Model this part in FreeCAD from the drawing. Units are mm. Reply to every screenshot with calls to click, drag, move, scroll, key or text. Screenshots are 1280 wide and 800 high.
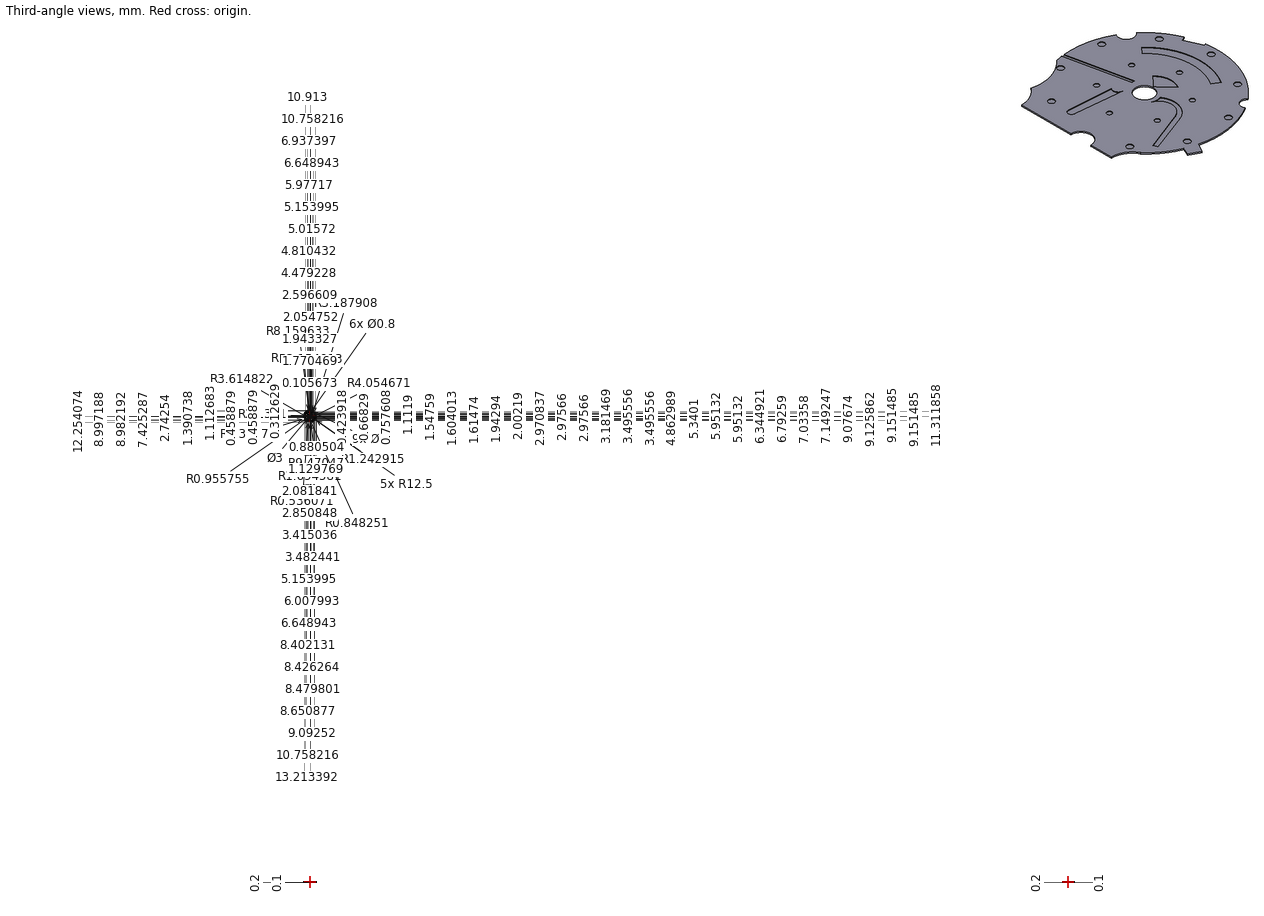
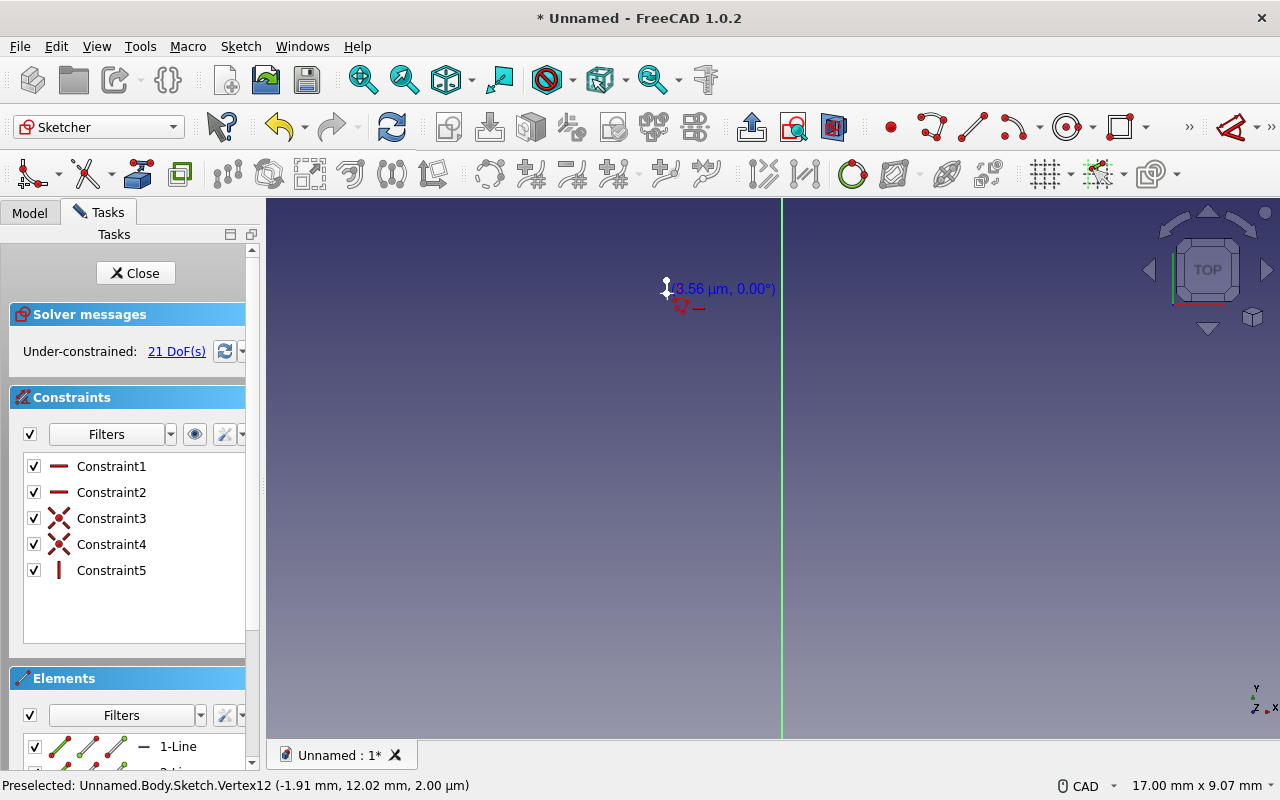
scroll(668, 292, down, 7)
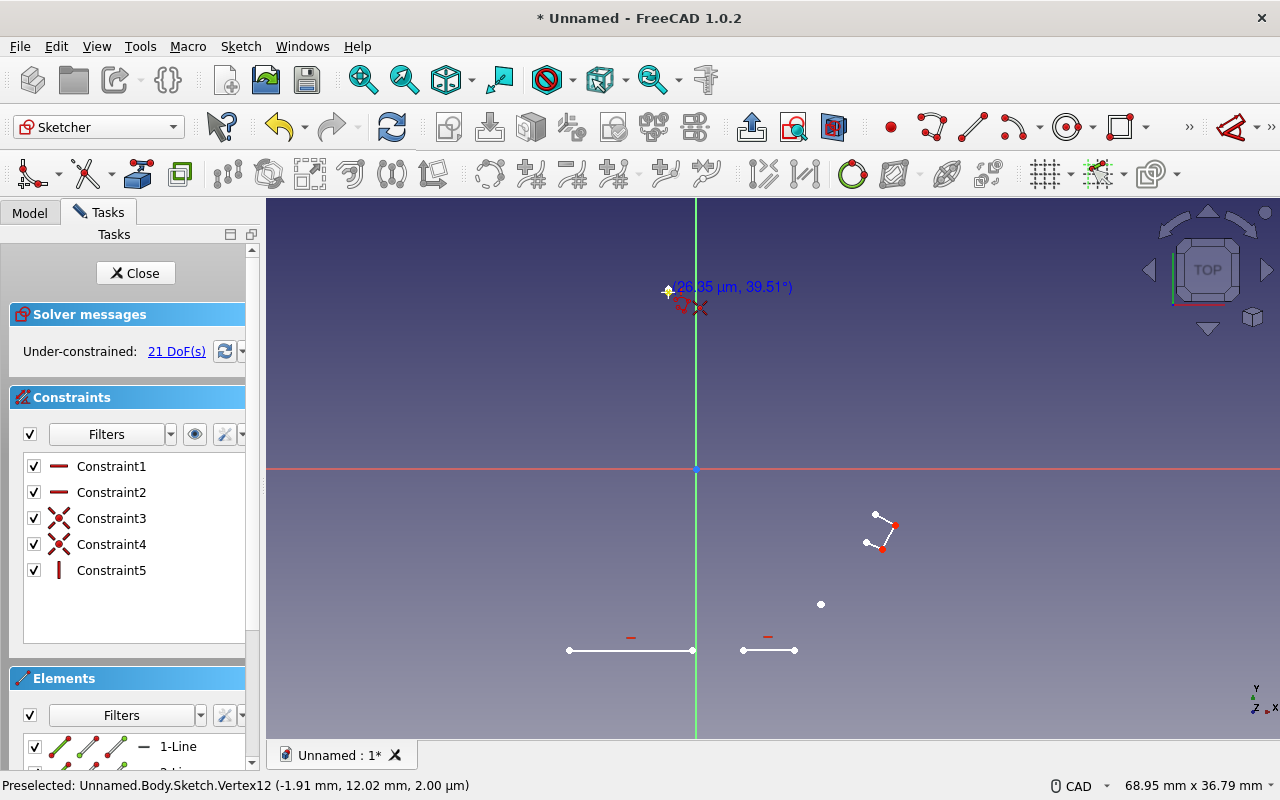
click(630, 309)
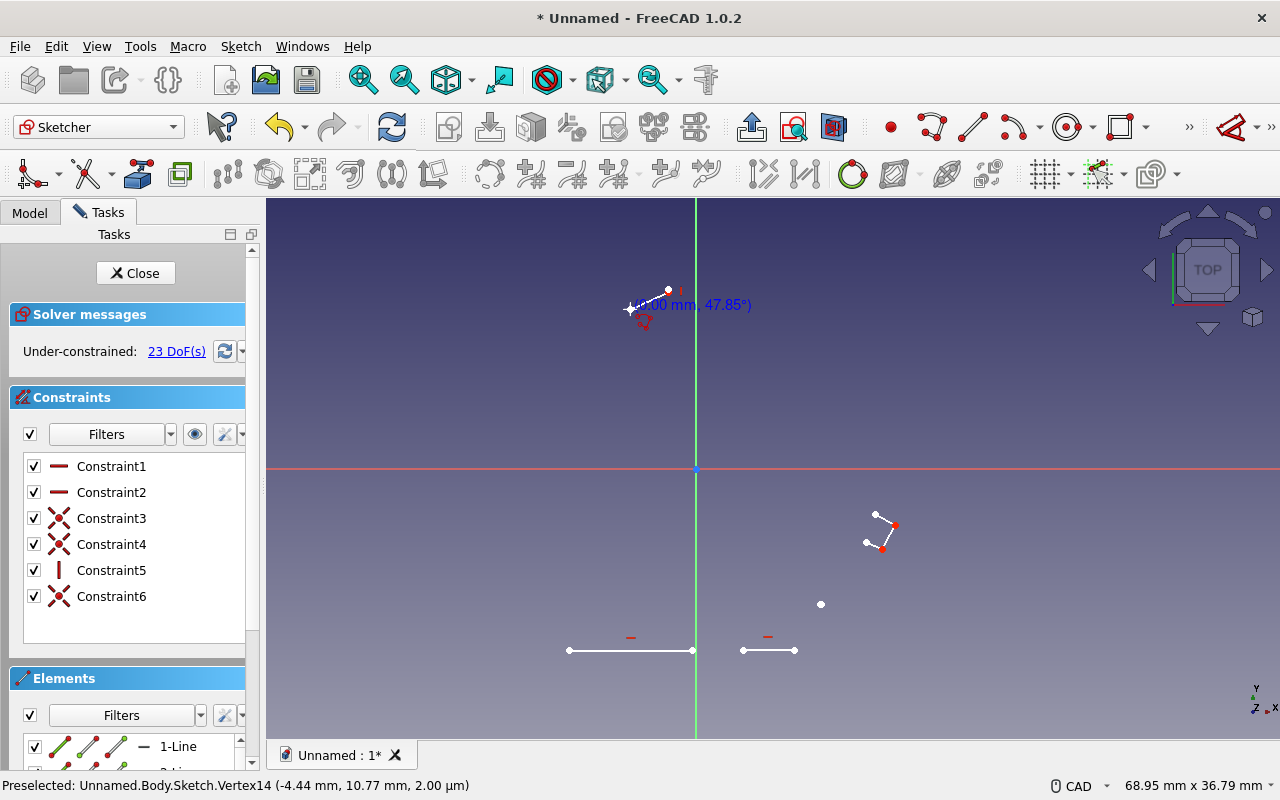
scroll(626, 300, up, 3)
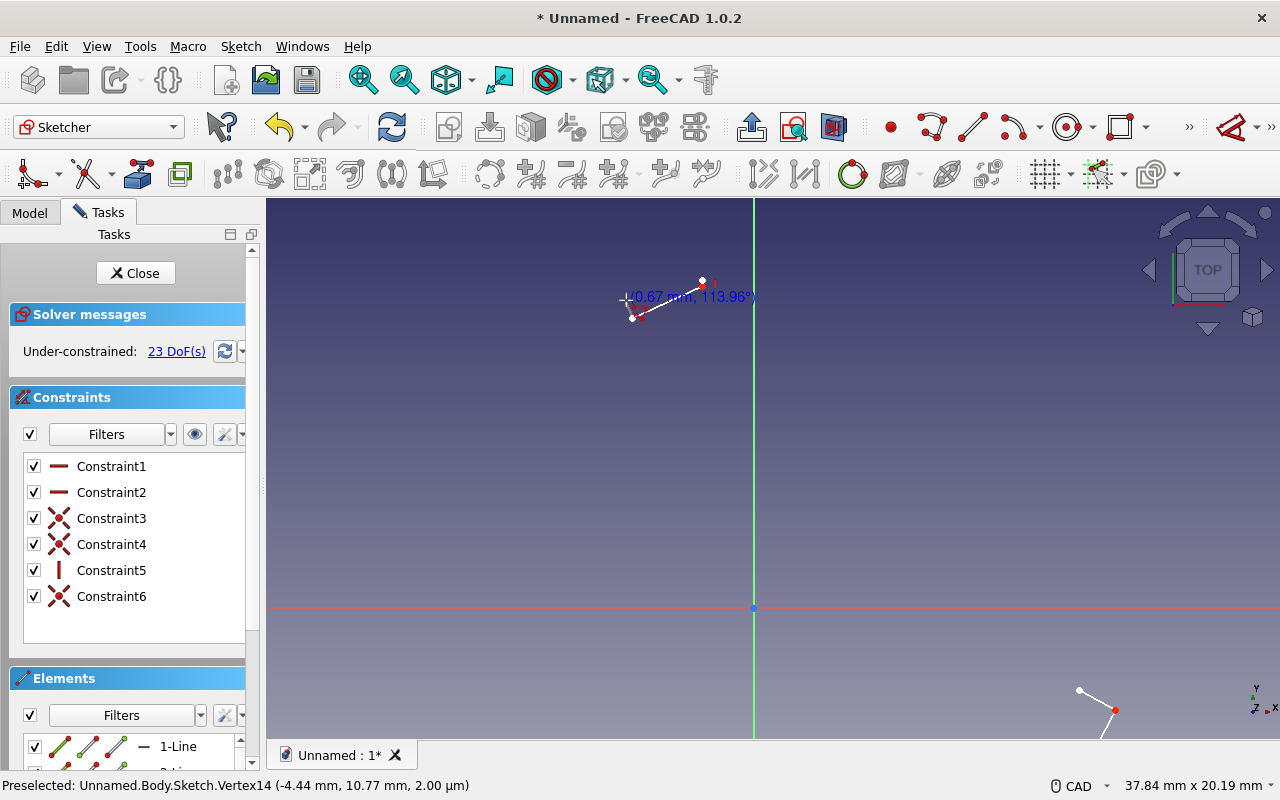
click(625, 299)
right_click(625, 299)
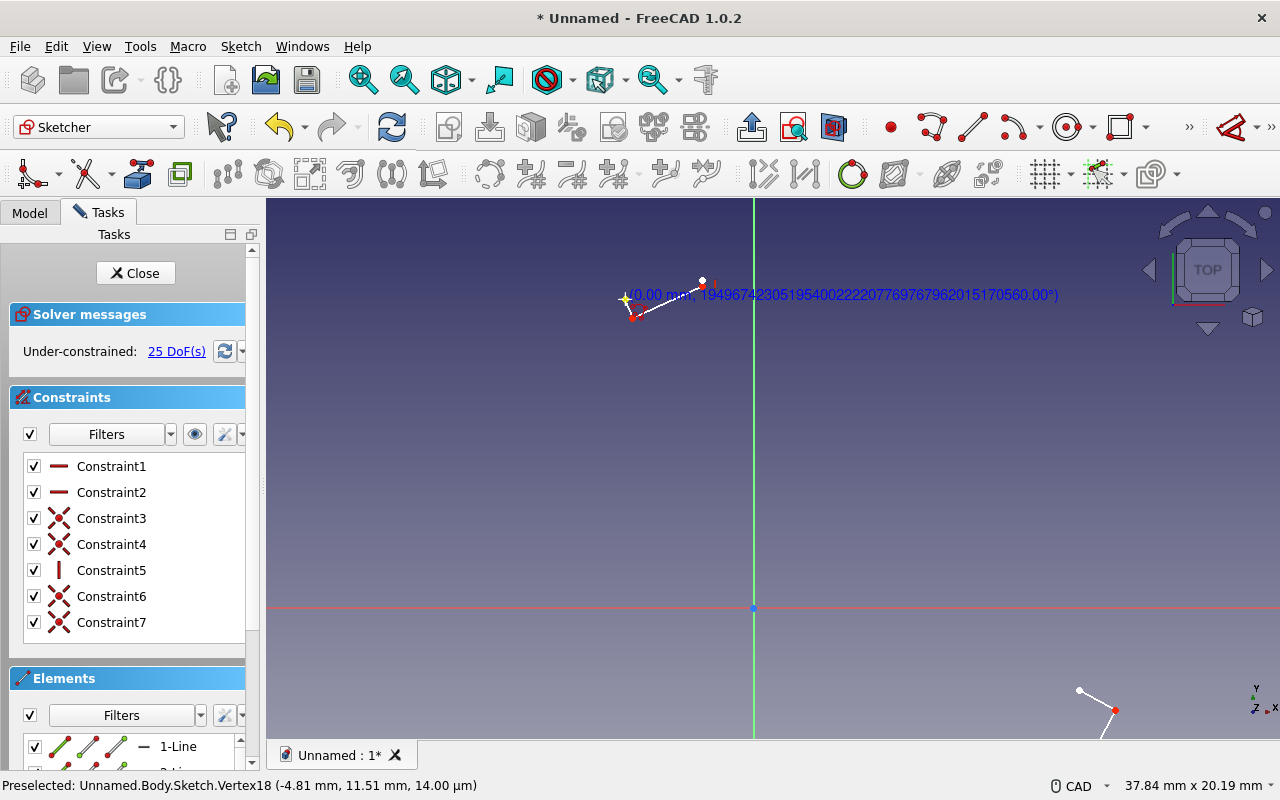
click(1040, 128)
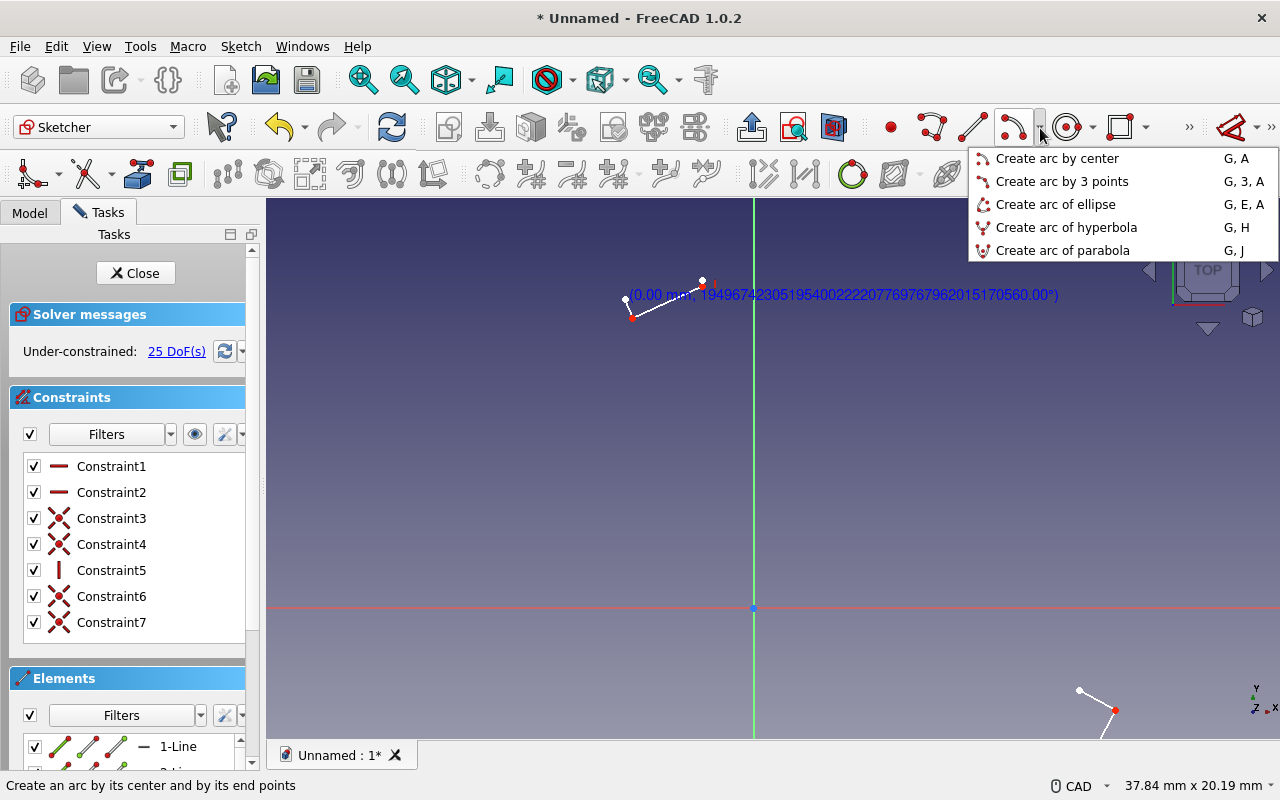
click(1124, 182)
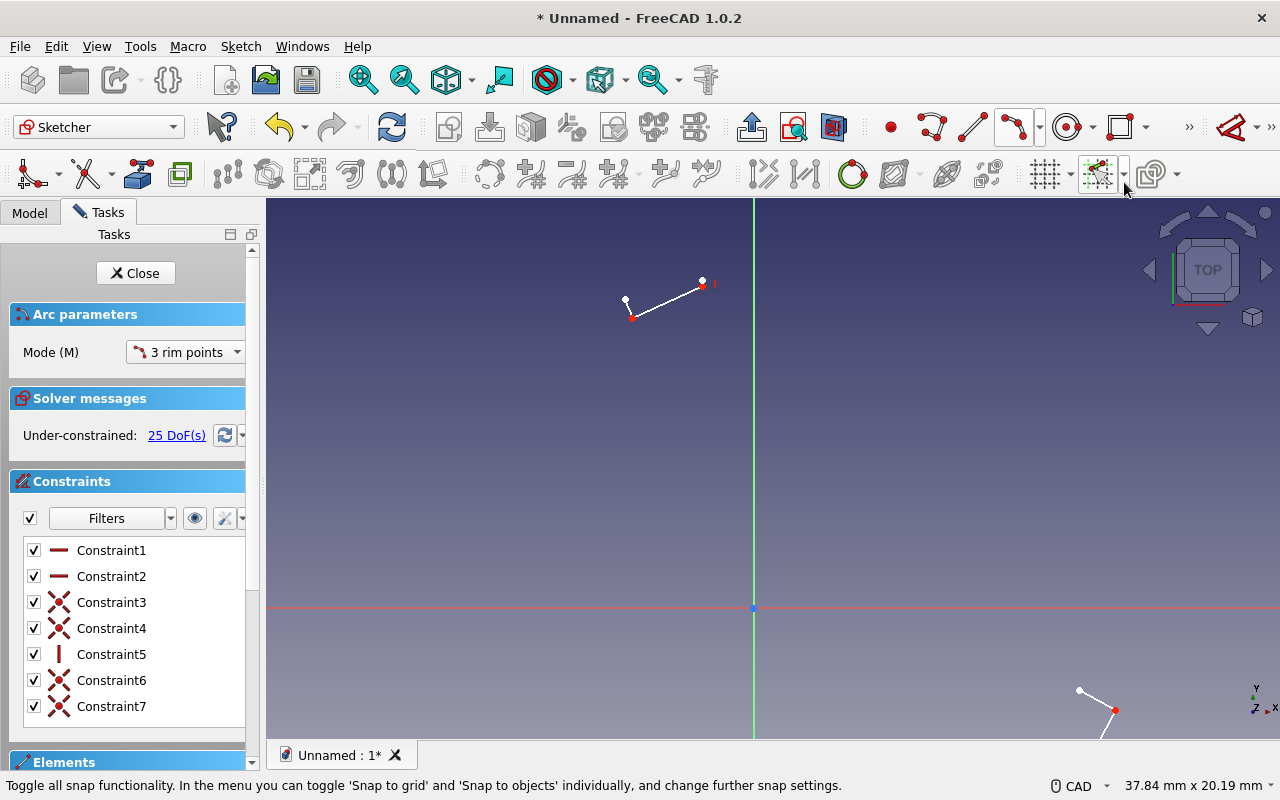
scroll(626, 300, down, 3)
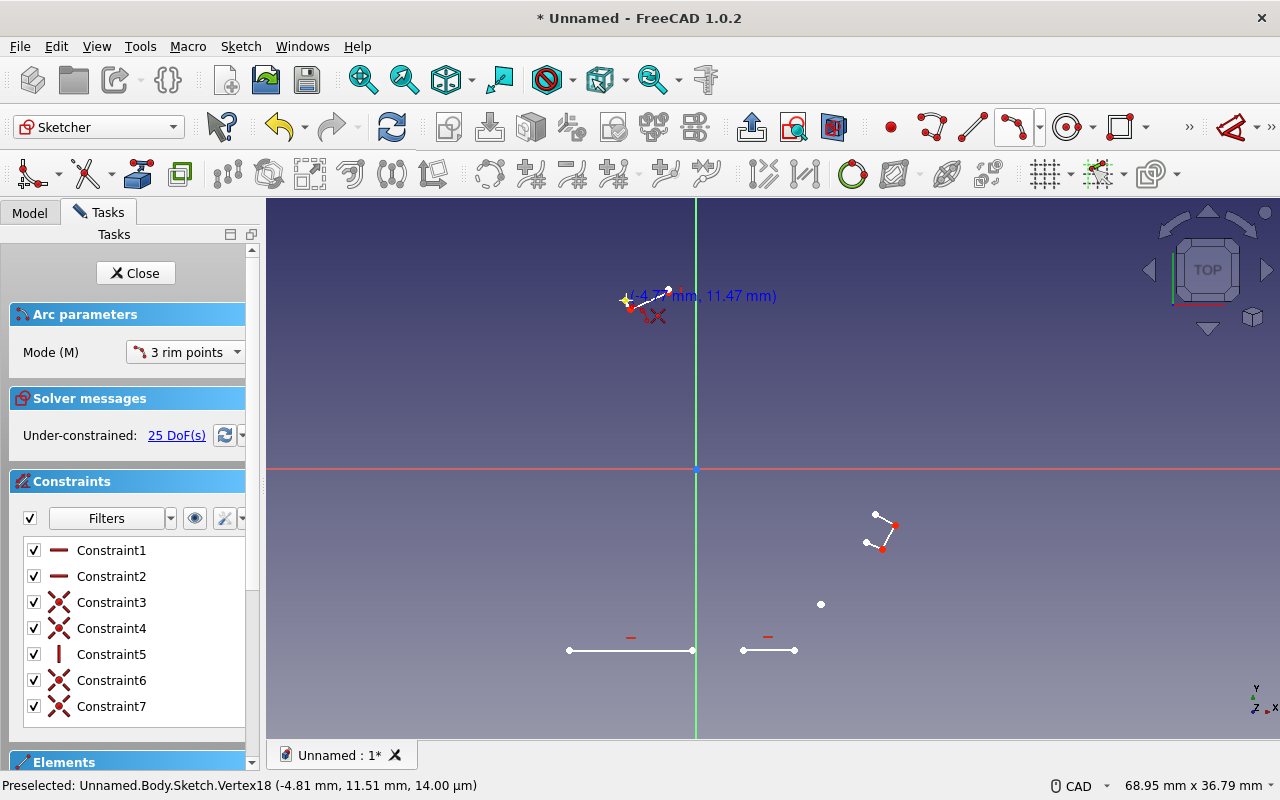
scroll(693, 650, up, 8)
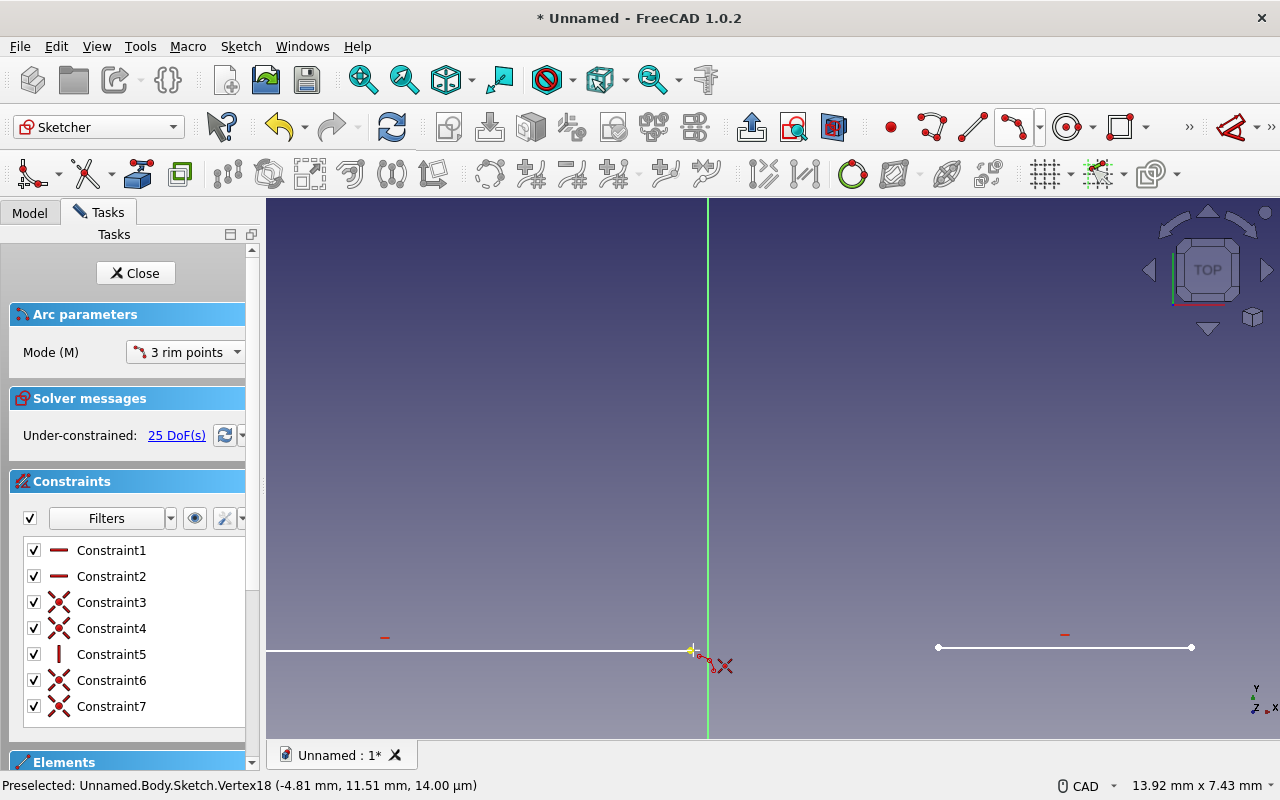
click(690, 651)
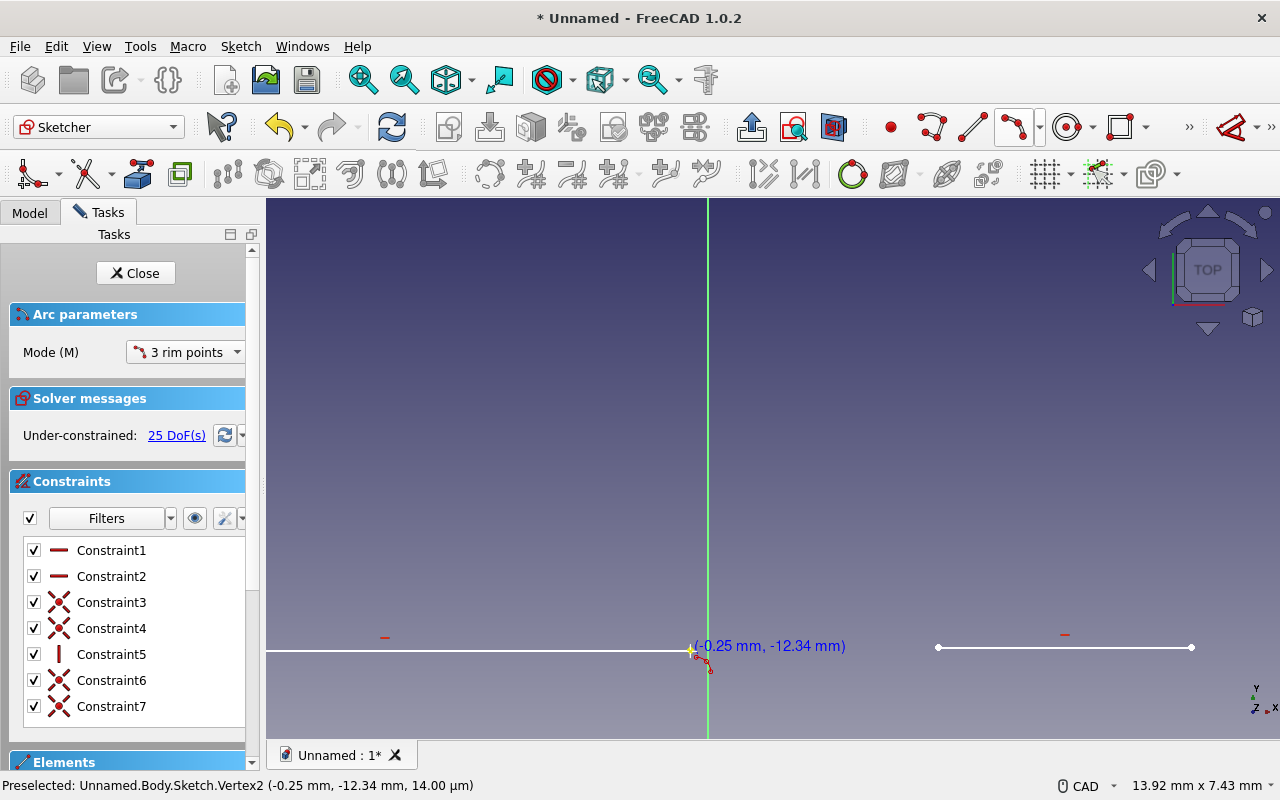
scroll(693, 651, down, 8)